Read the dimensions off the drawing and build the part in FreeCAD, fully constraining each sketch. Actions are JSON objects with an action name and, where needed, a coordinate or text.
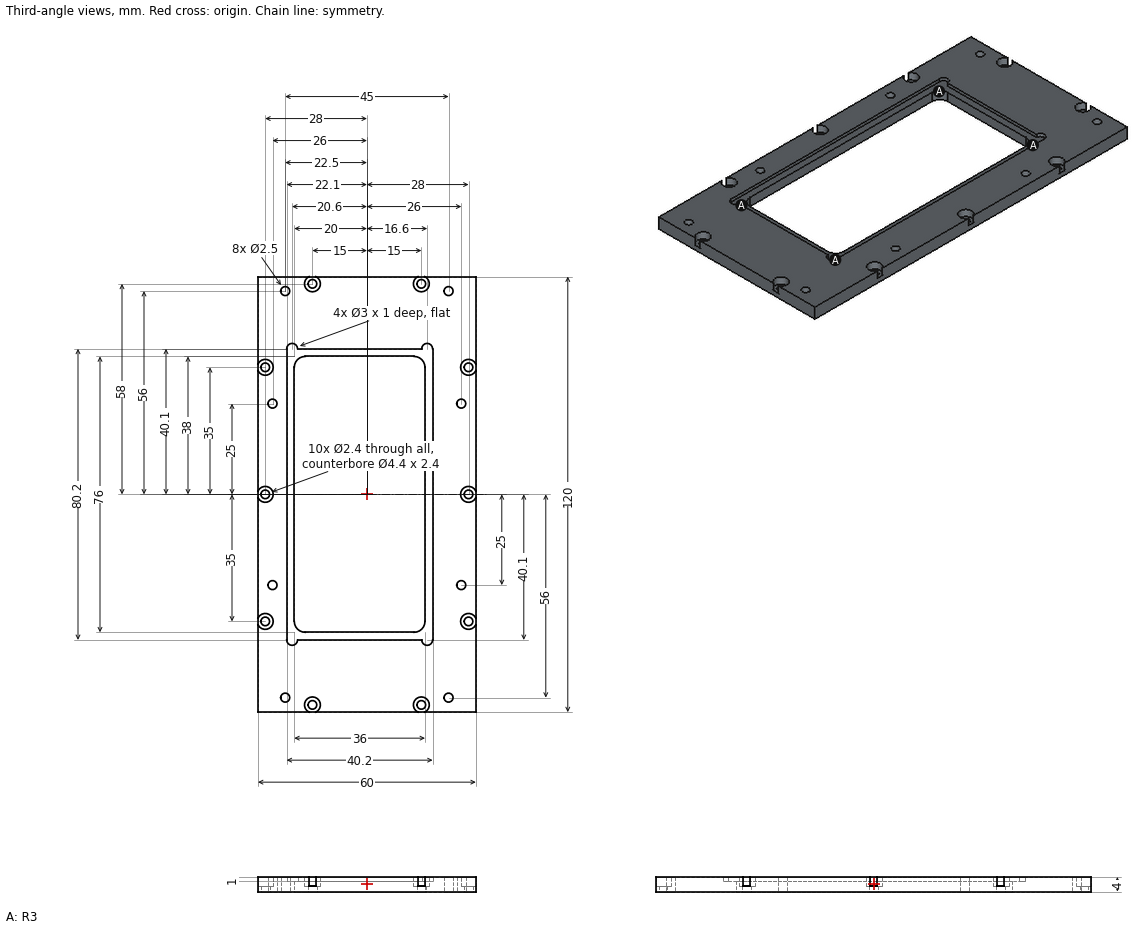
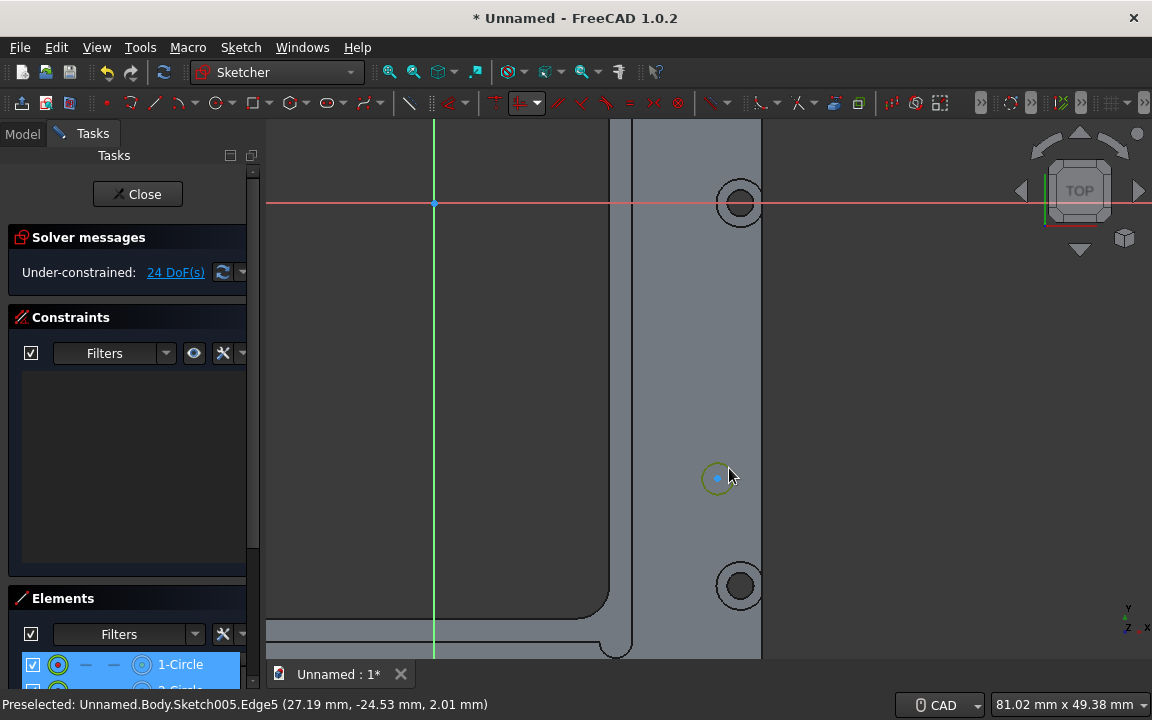
{"action": "scroll", "coordinate": [729, 469], "scroll_direction": "down", "scroll_amount": 6}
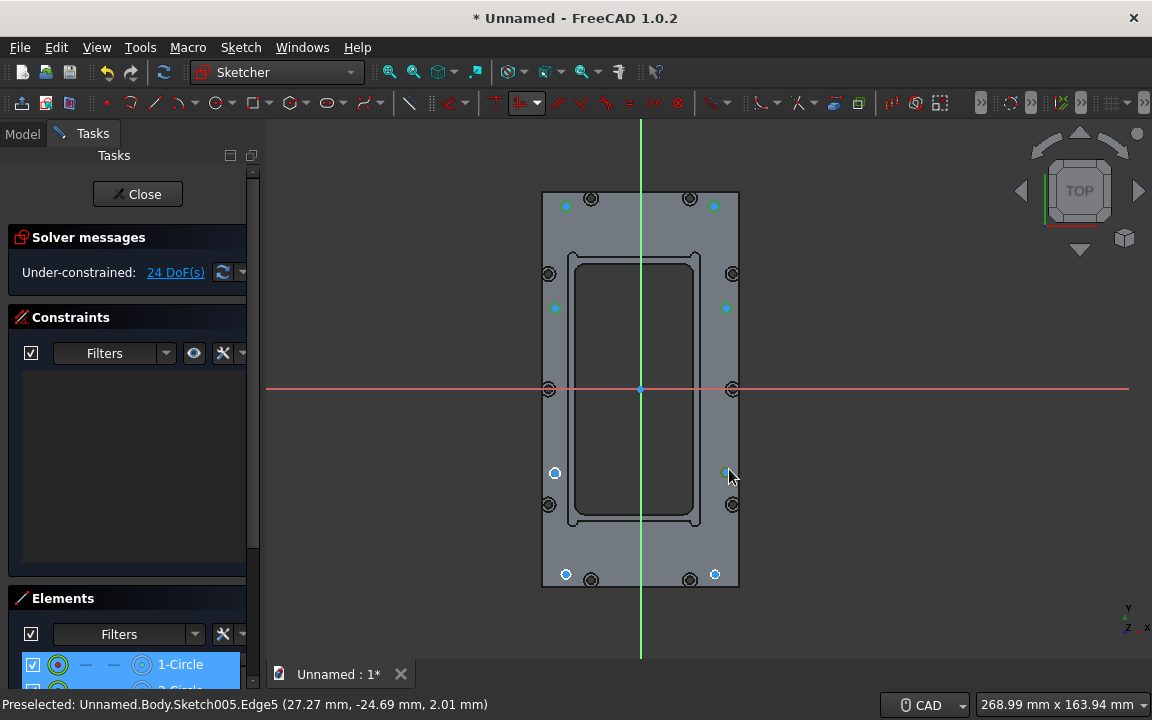
{"action": "scroll", "coordinate": [559, 470], "scroll_direction": "up", "scroll_amount": 6}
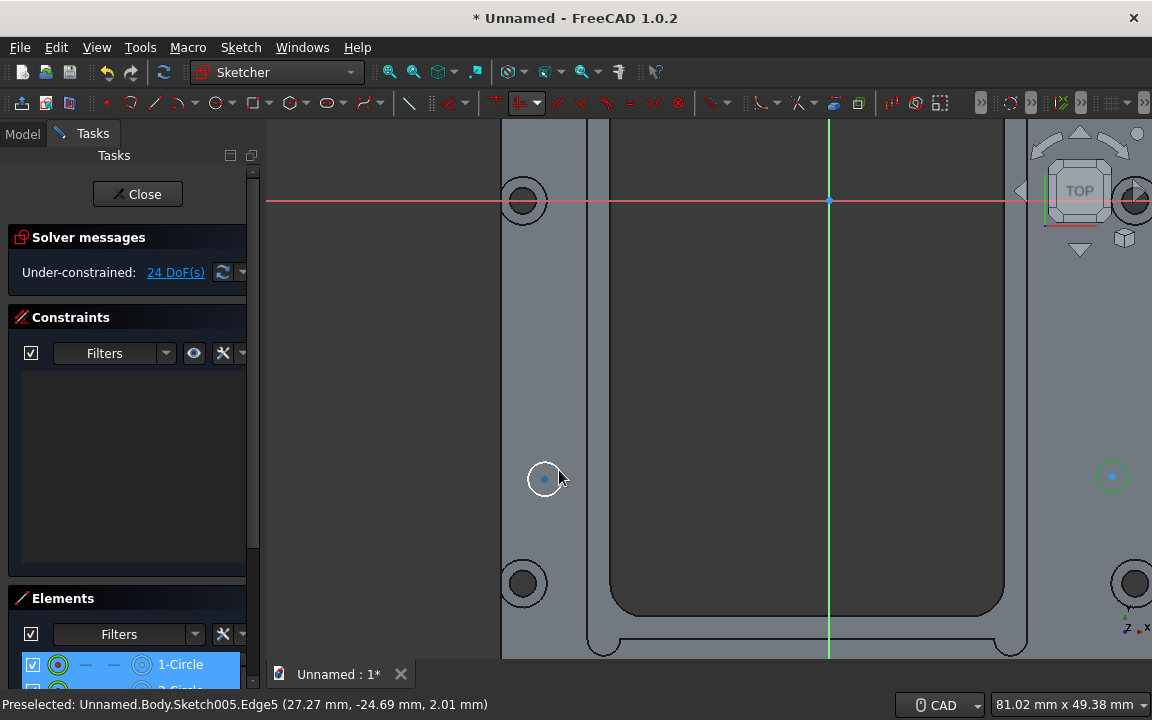
{"action": "left_click", "coordinate": [557, 467]}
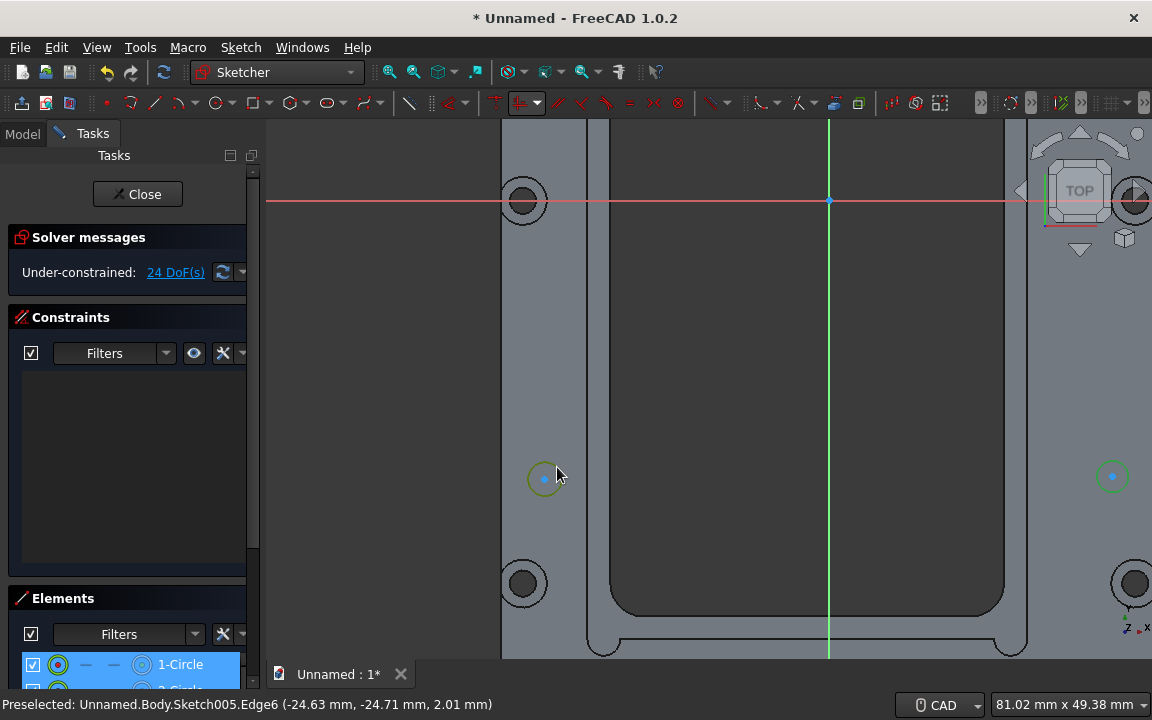
{"action": "scroll", "coordinate": [559, 470], "scroll_direction": "down", "scroll_amount": 6}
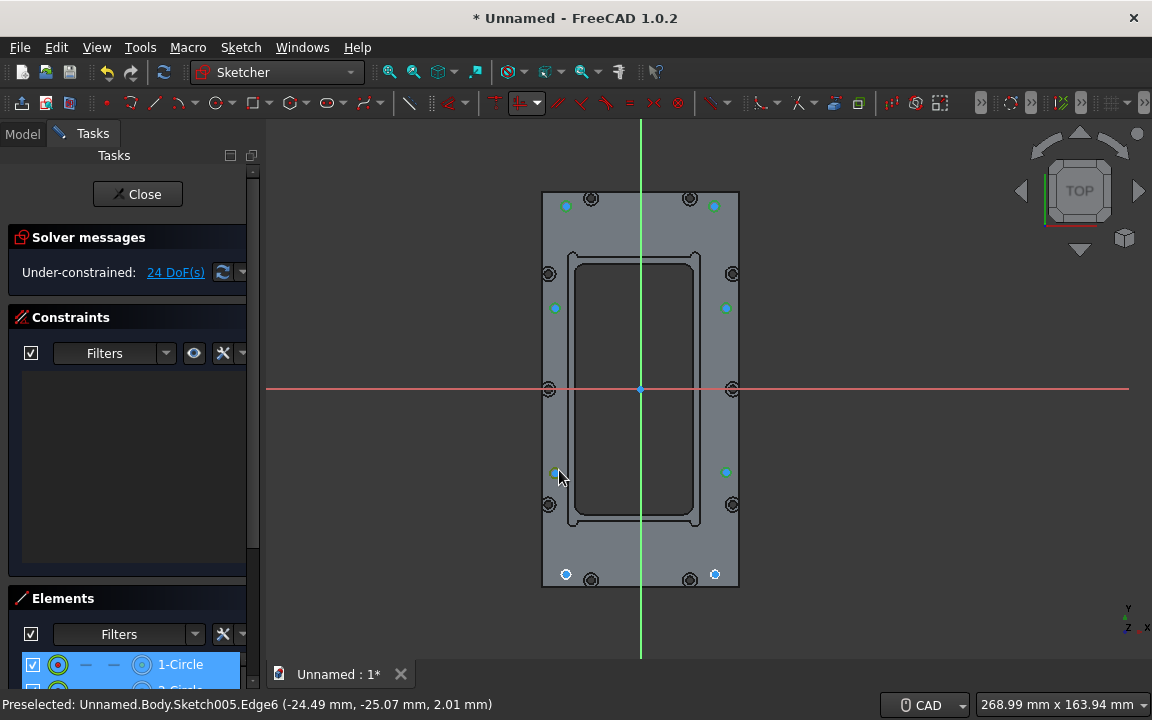
{"action": "scroll", "coordinate": [718, 571], "scroll_direction": "up", "scroll_amount": 7}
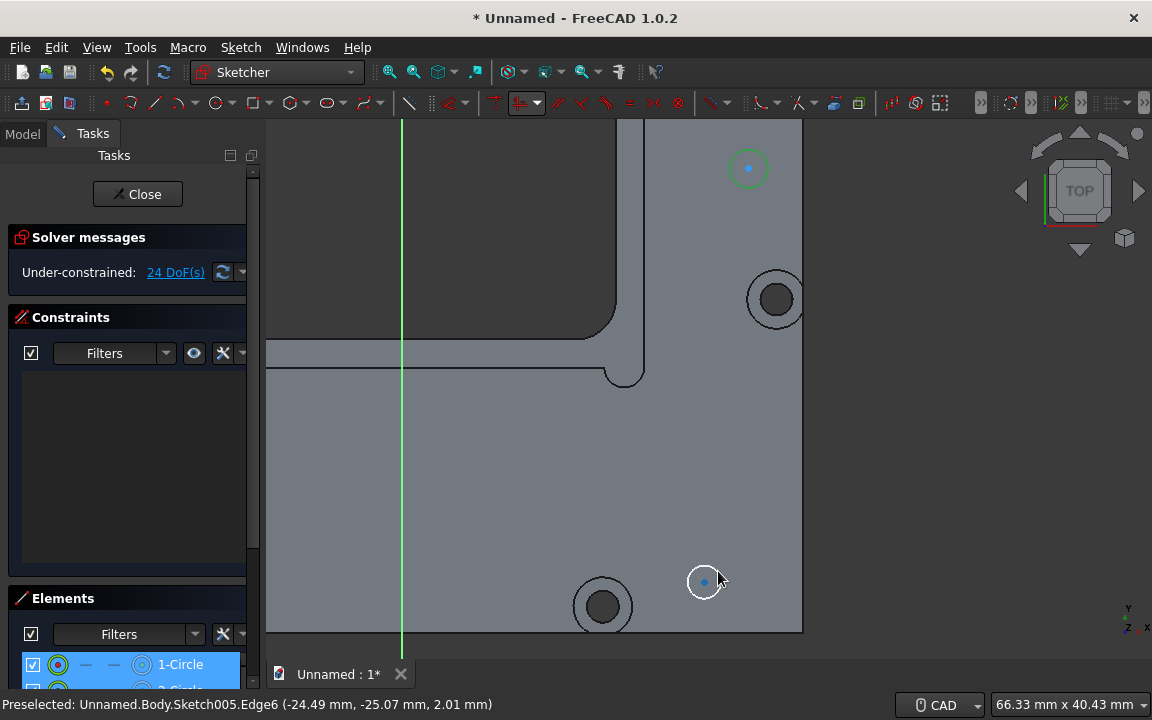
{"action": "left_click", "coordinate": [716, 570]}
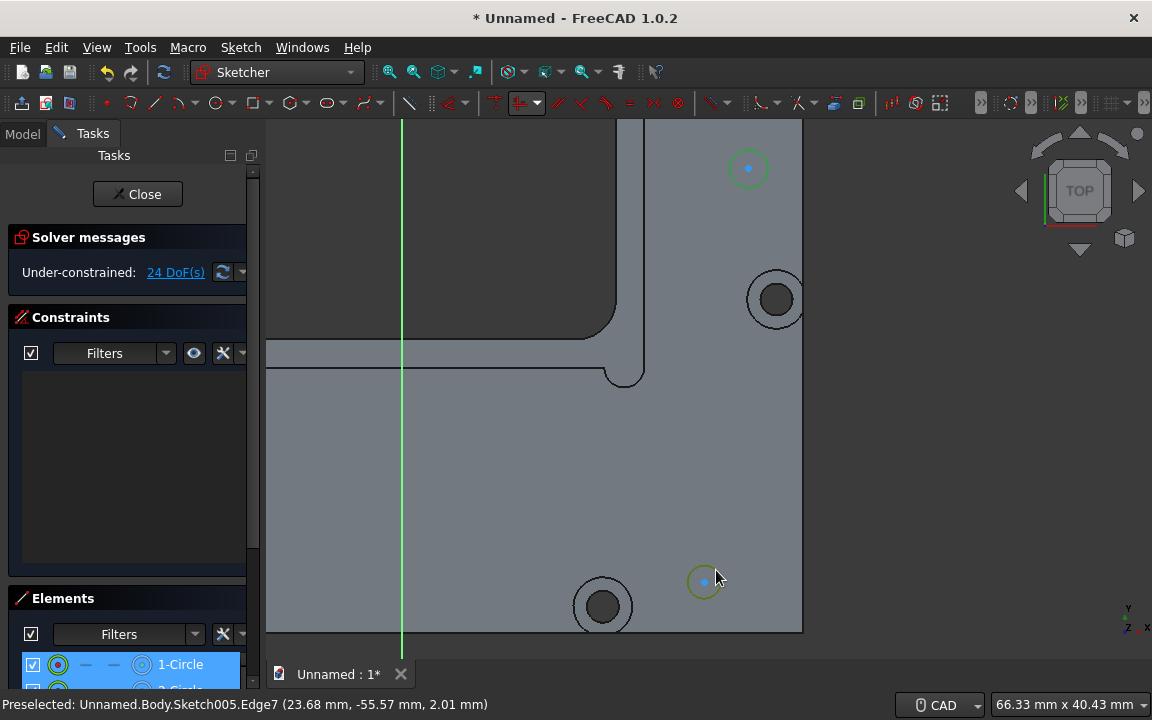
{"action": "scroll", "coordinate": [718, 571], "scroll_direction": "down", "scroll_amount": 7}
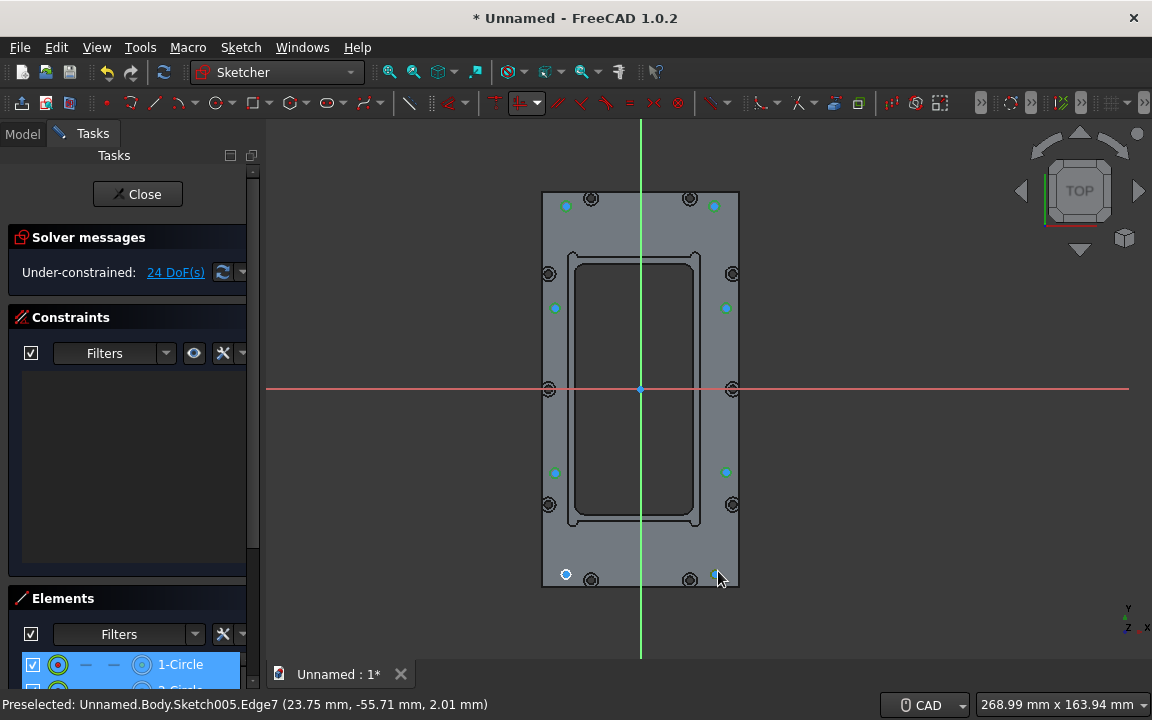
{"action": "scroll", "coordinate": [569, 571], "scroll_direction": "up", "scroll_amount": 6}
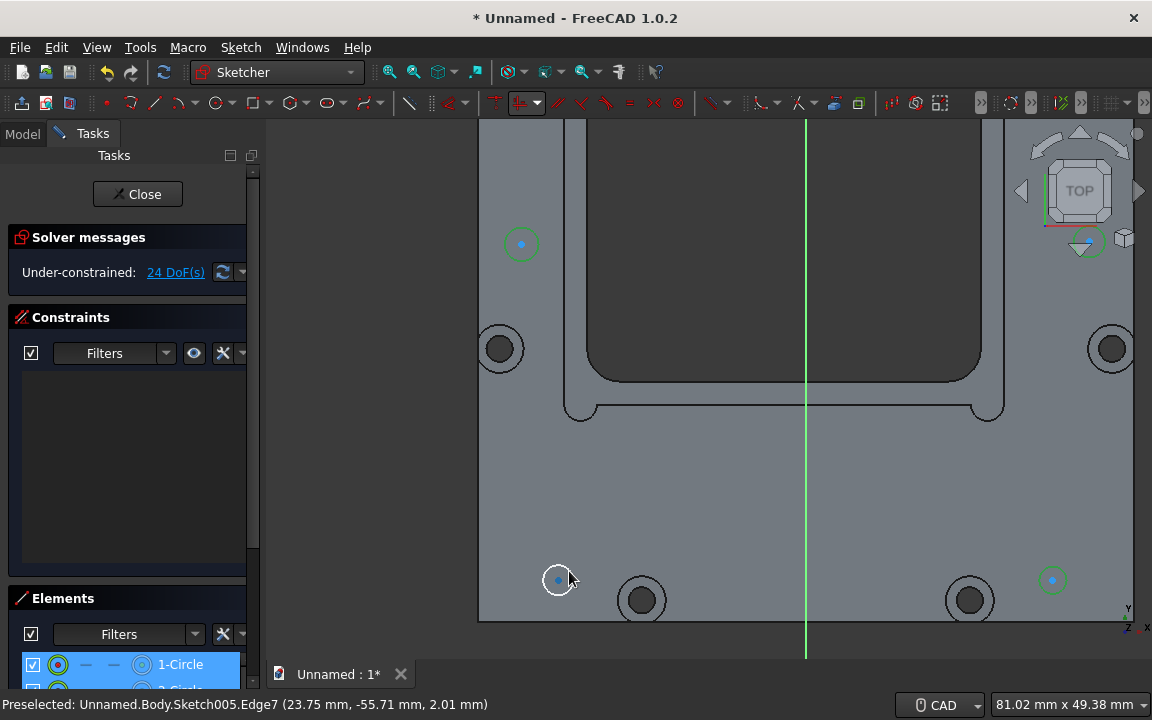
{"action": "left_click", "coordinate": [569, 570]}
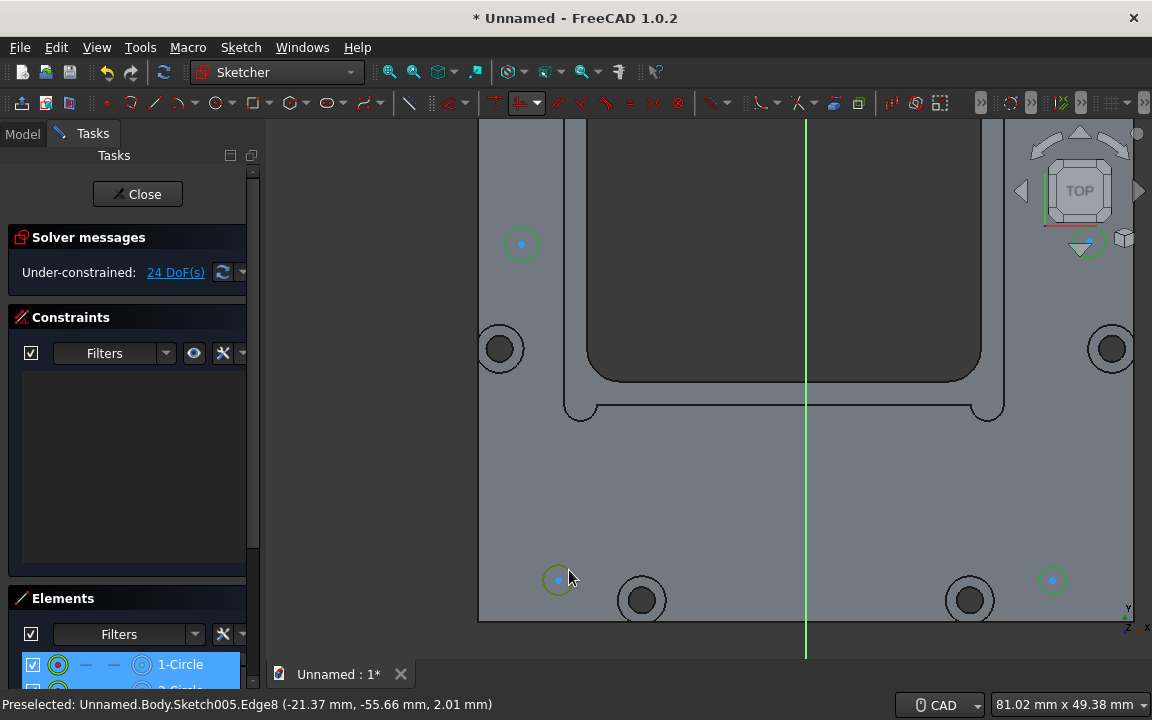
{"action": "left_click", "coordinate": [630, 104]}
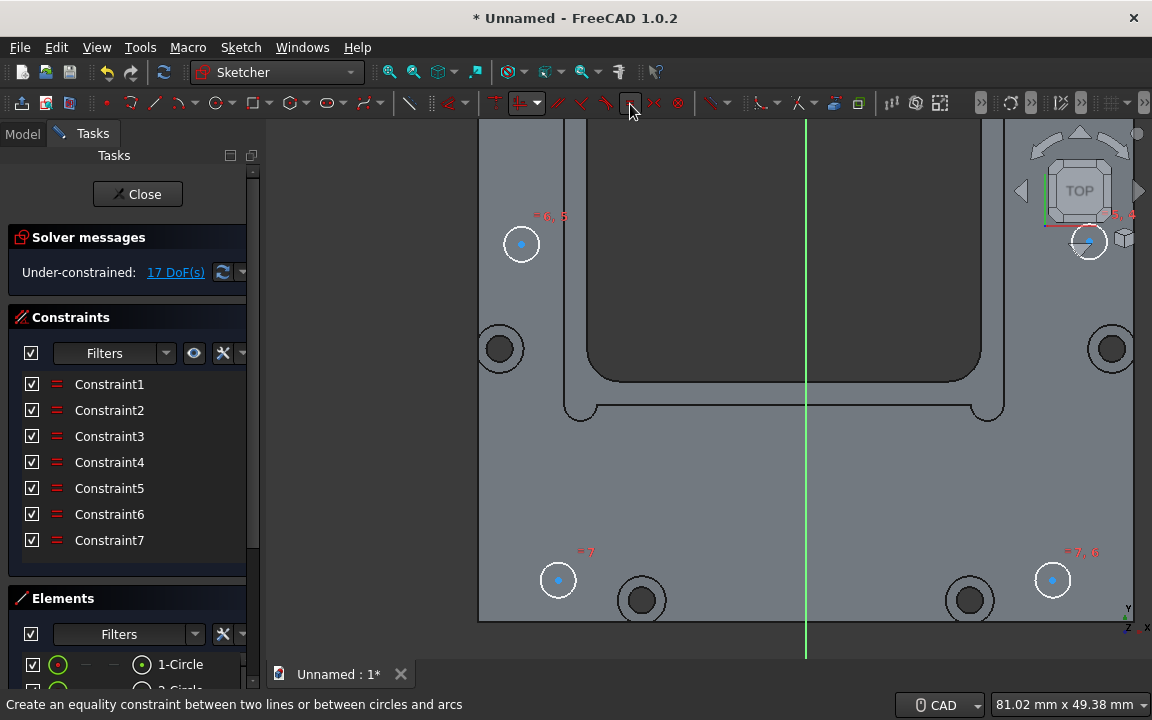
{"action": "scroll", "coordinate": [569, 571], "scroll_direction": "down", "scroll_amount": 6}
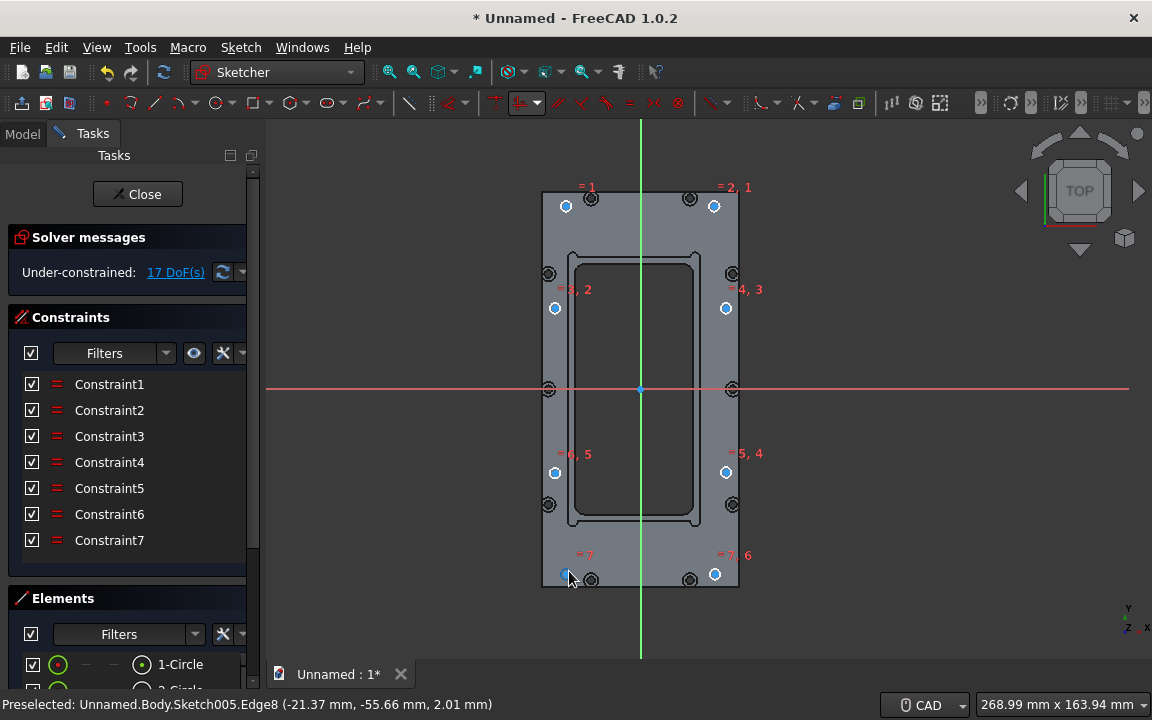
{"action": "left_click", "coordinate": [566, 206]}